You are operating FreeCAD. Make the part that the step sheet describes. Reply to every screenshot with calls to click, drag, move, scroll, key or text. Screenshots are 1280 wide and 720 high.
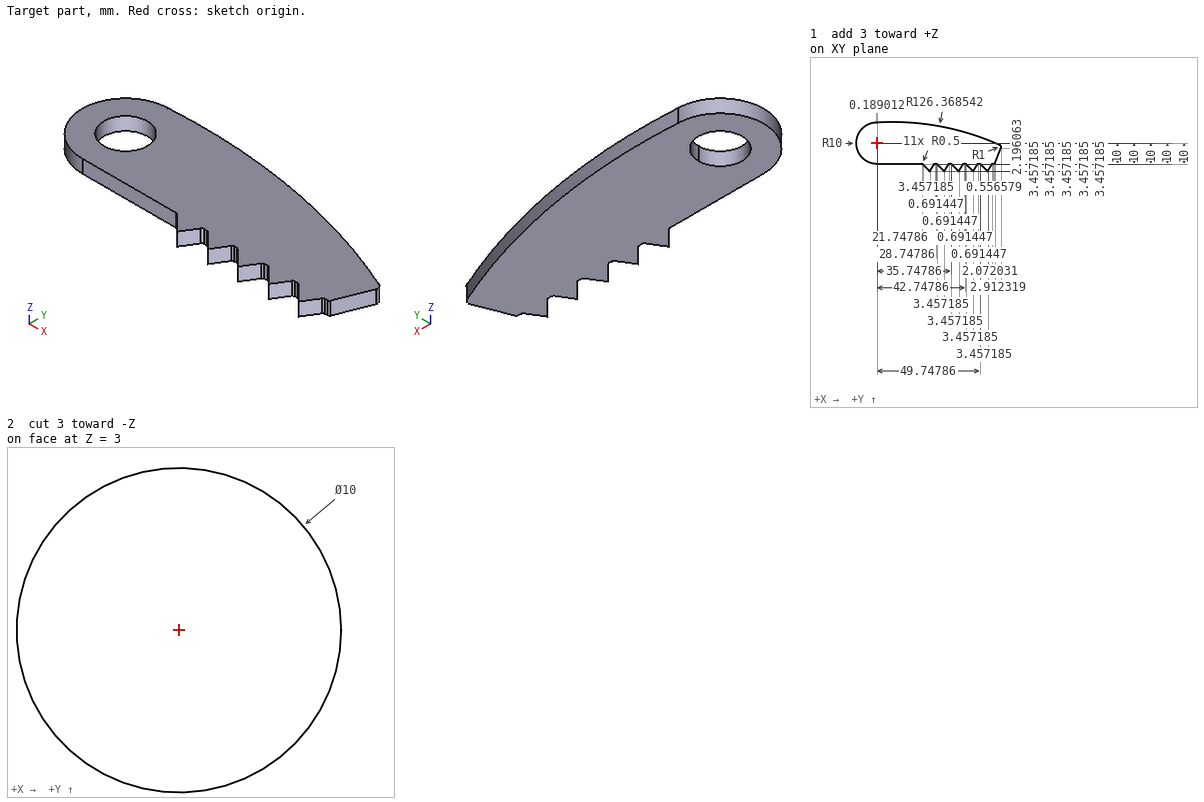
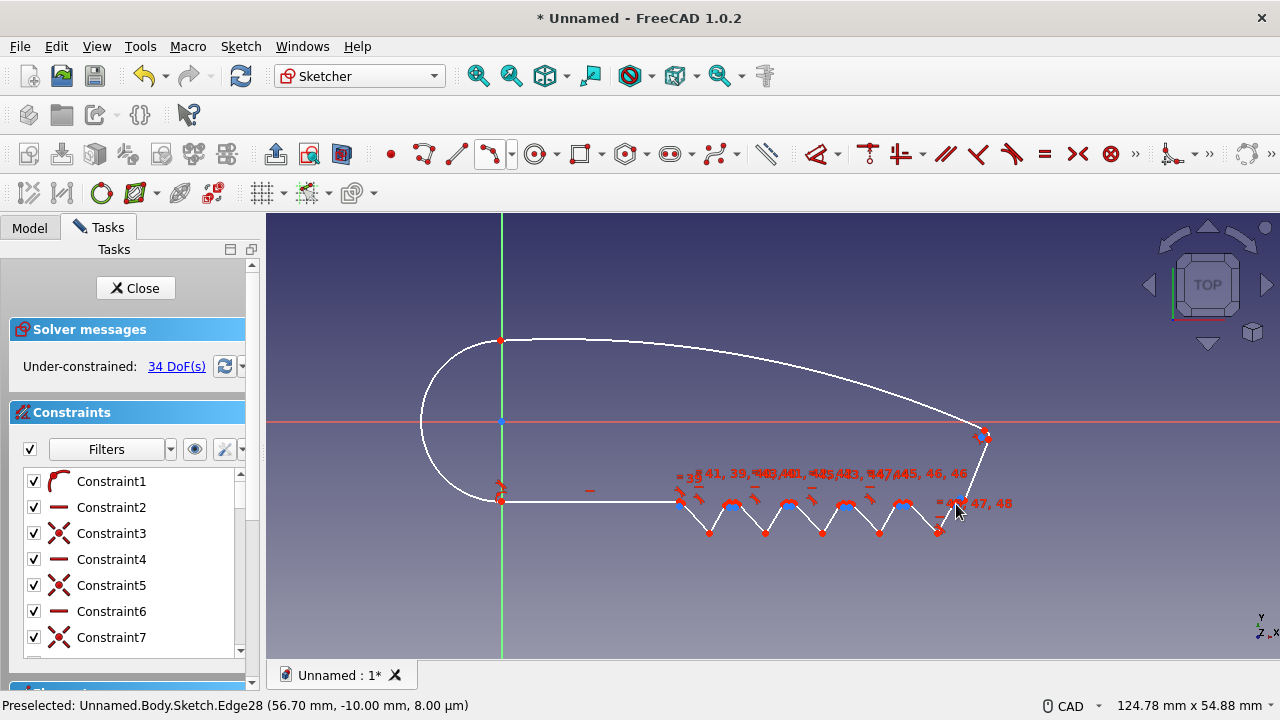
click(502, 421)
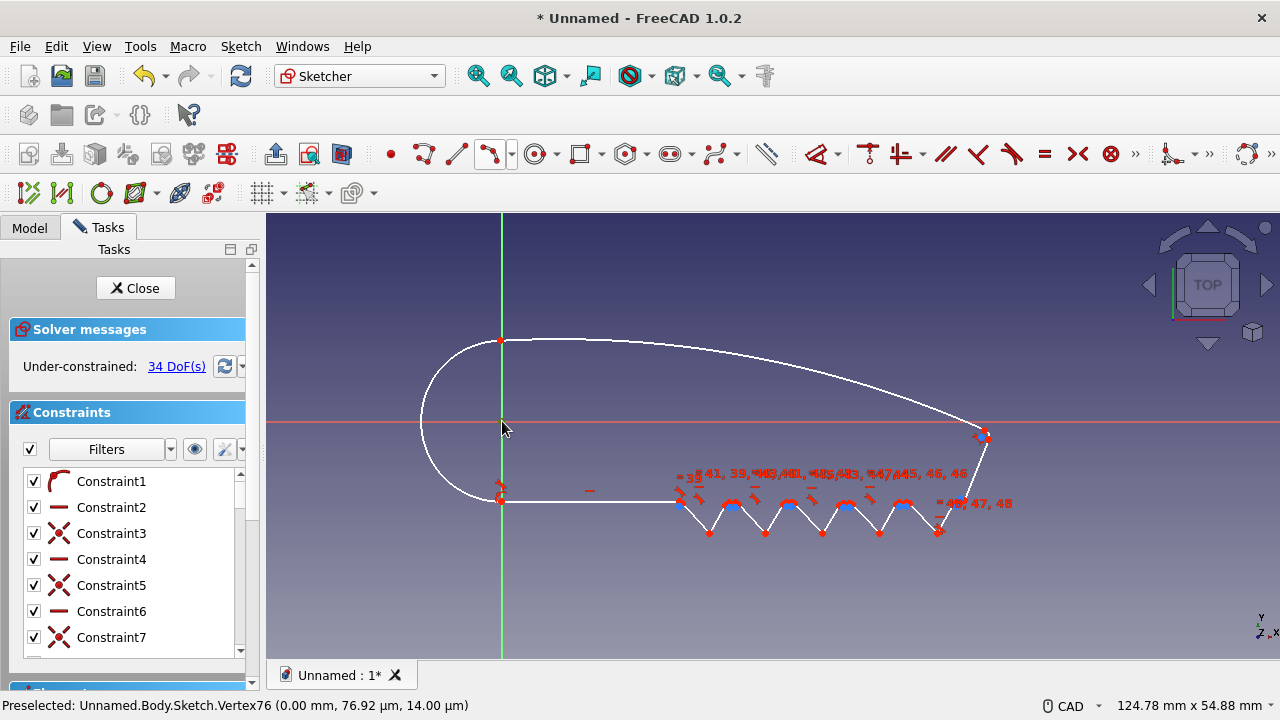
click(353, 422)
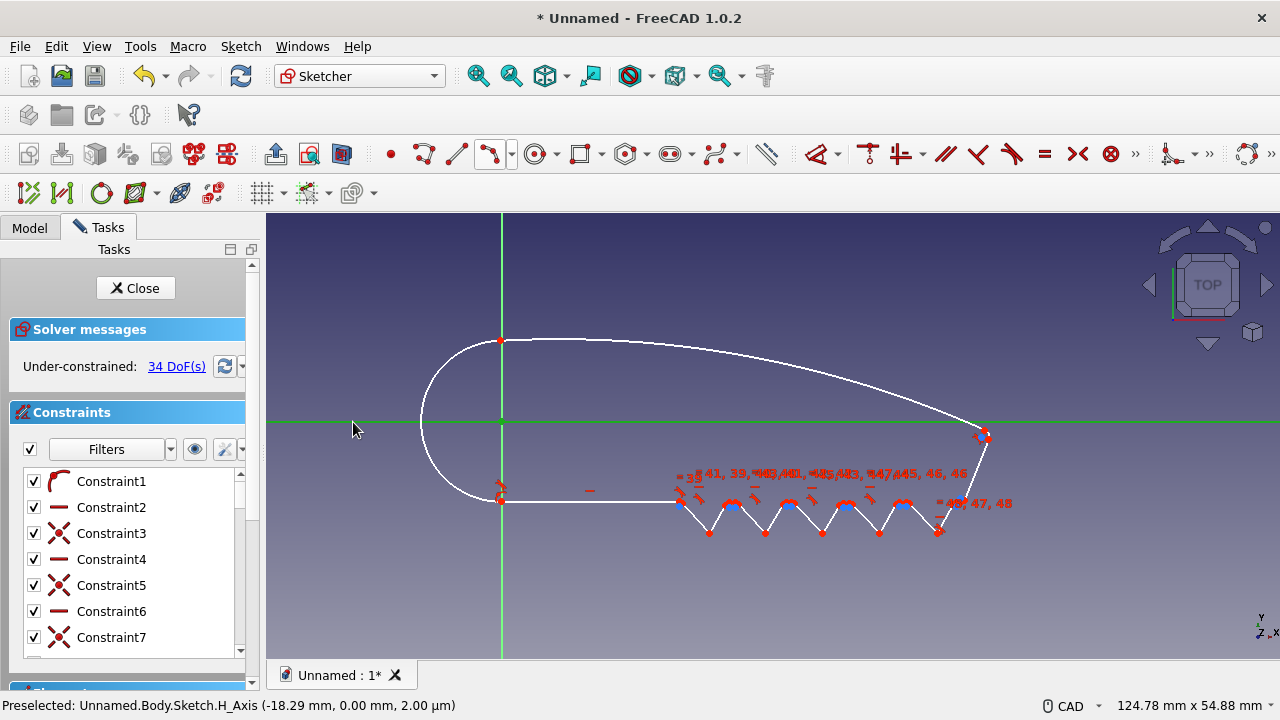
click(868, 154)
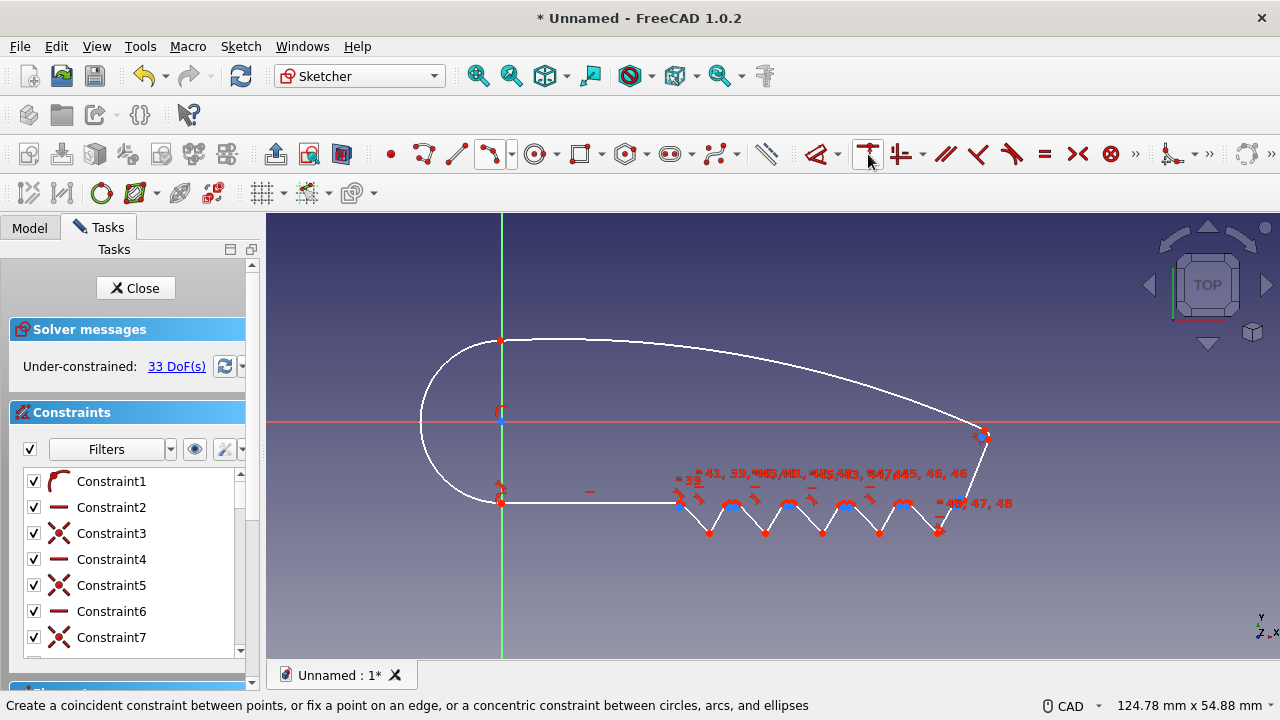
scroll(681, 503, up, 12)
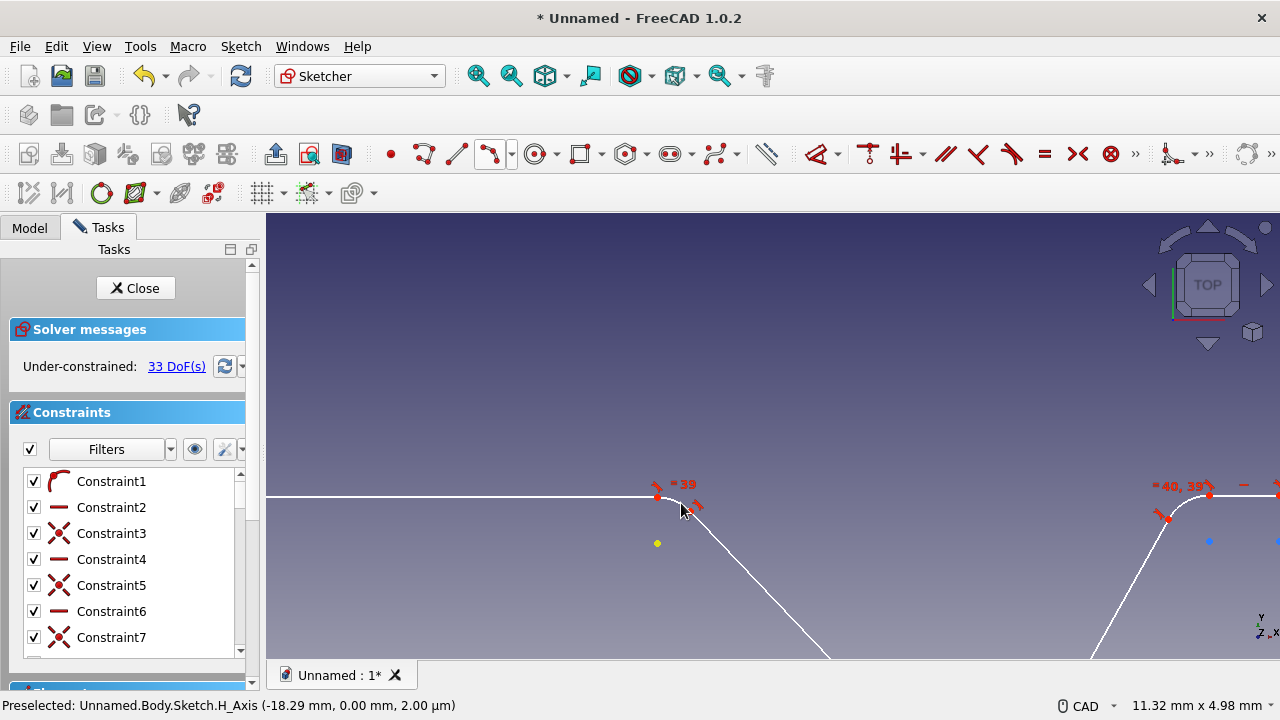
click(676, 501)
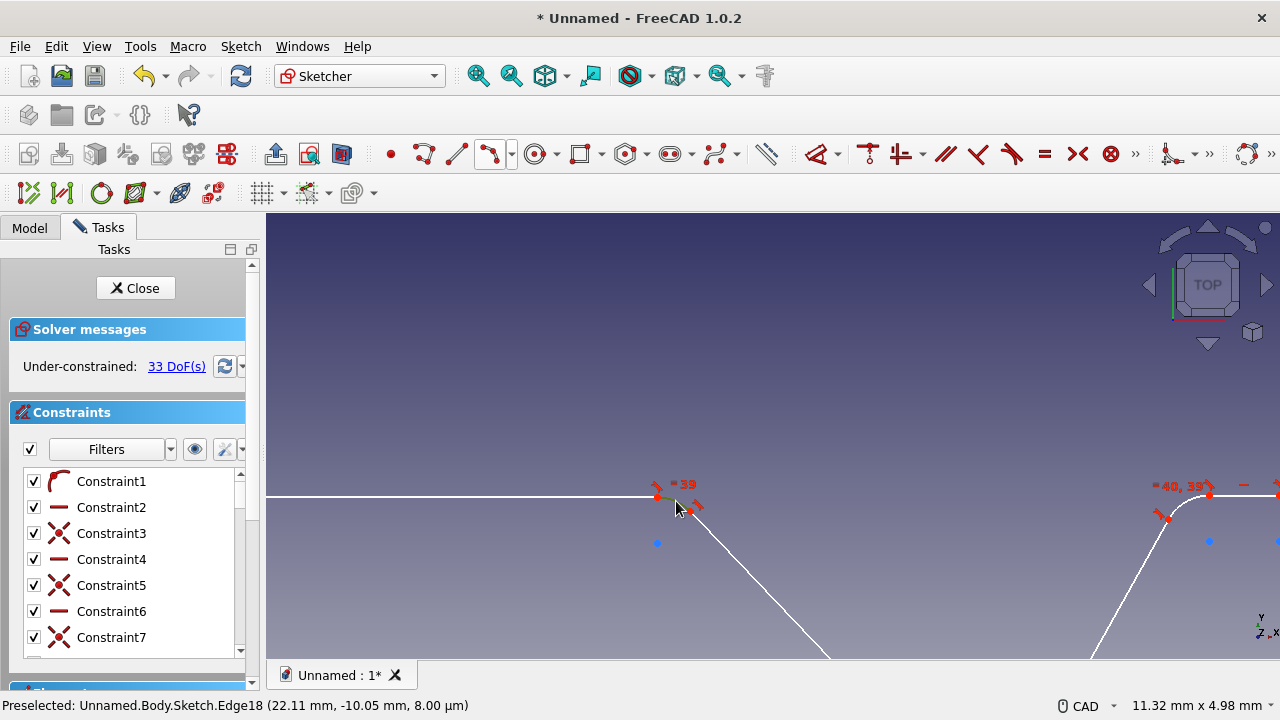
click(838, 154)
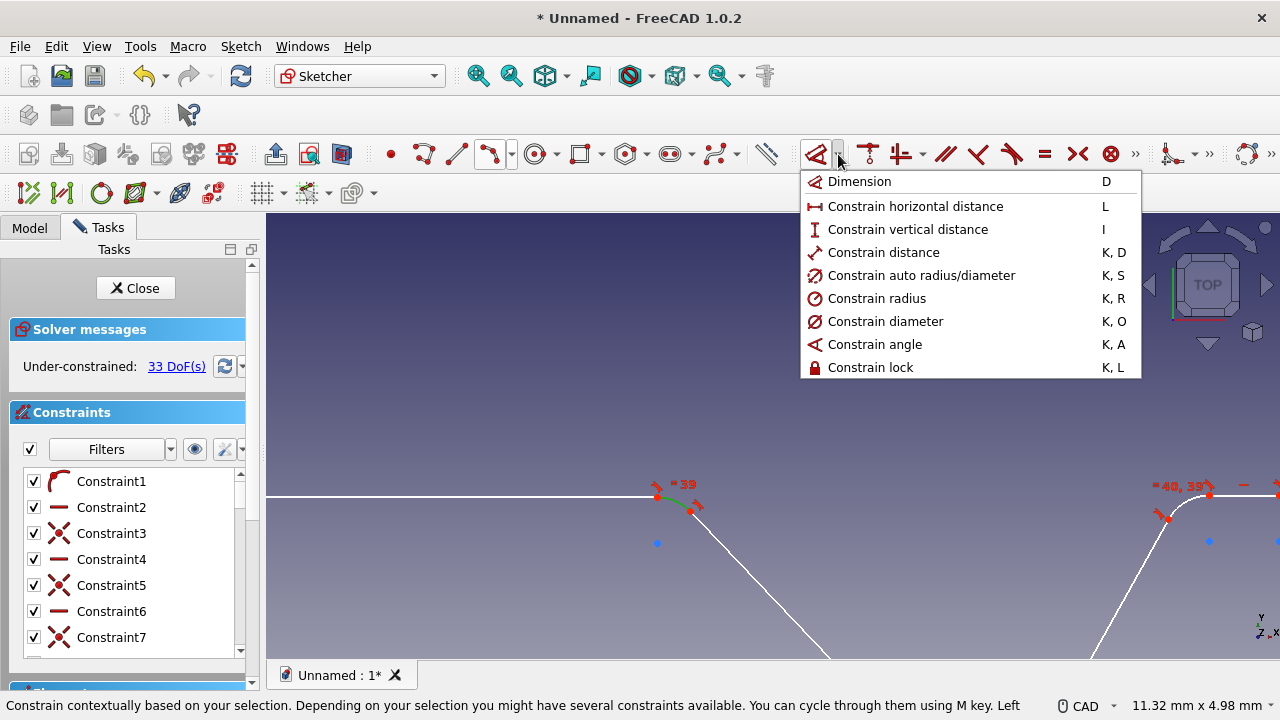
click(971, 298)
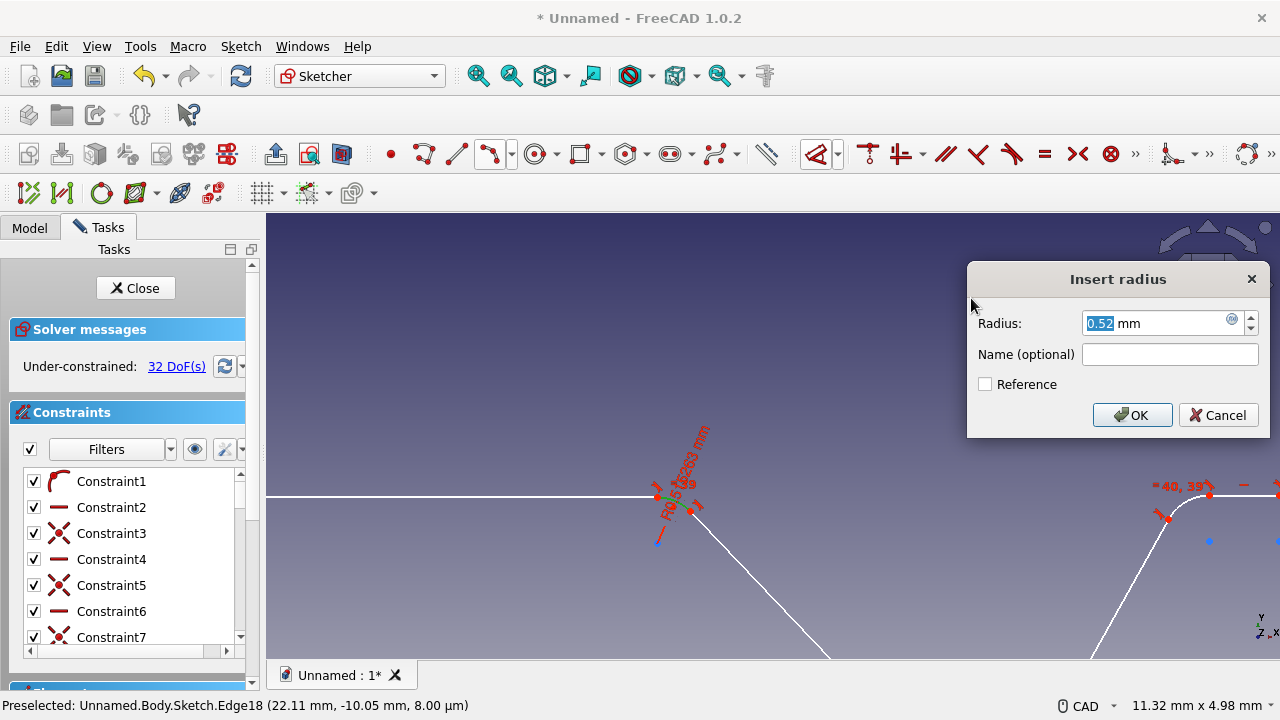
text(0.5)
key(Return)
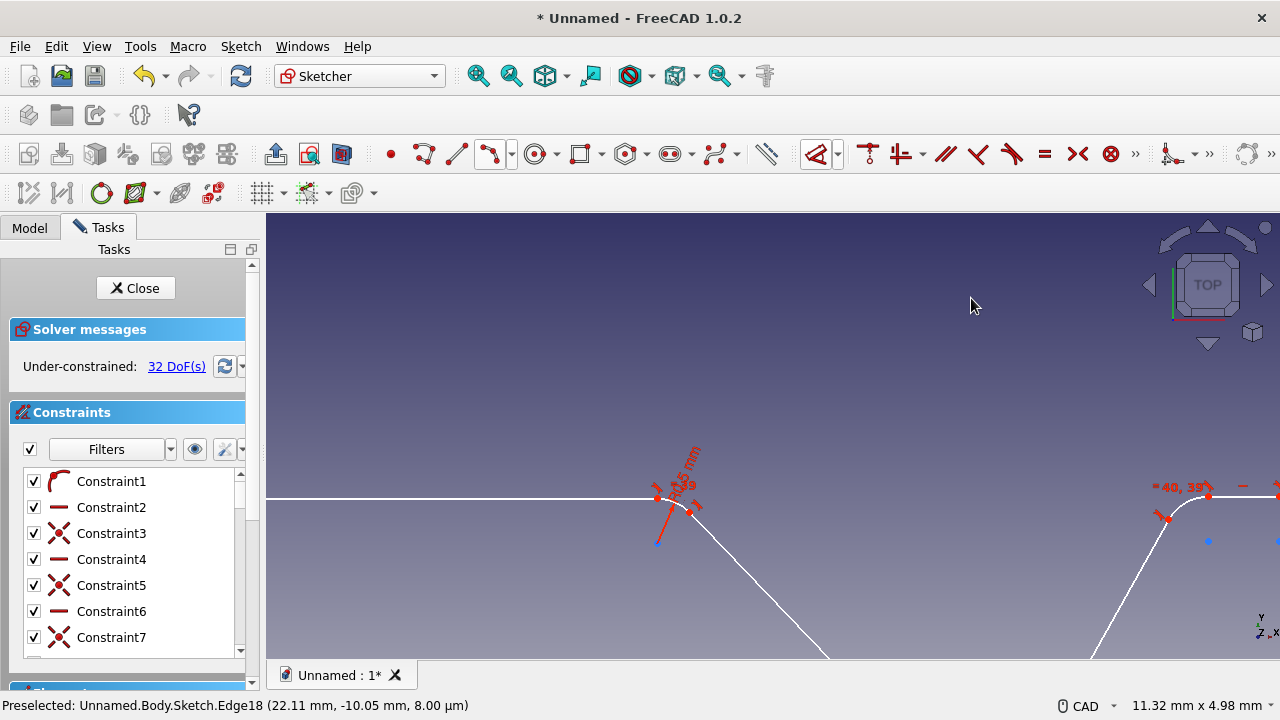
scroll(681, 503, down, 12)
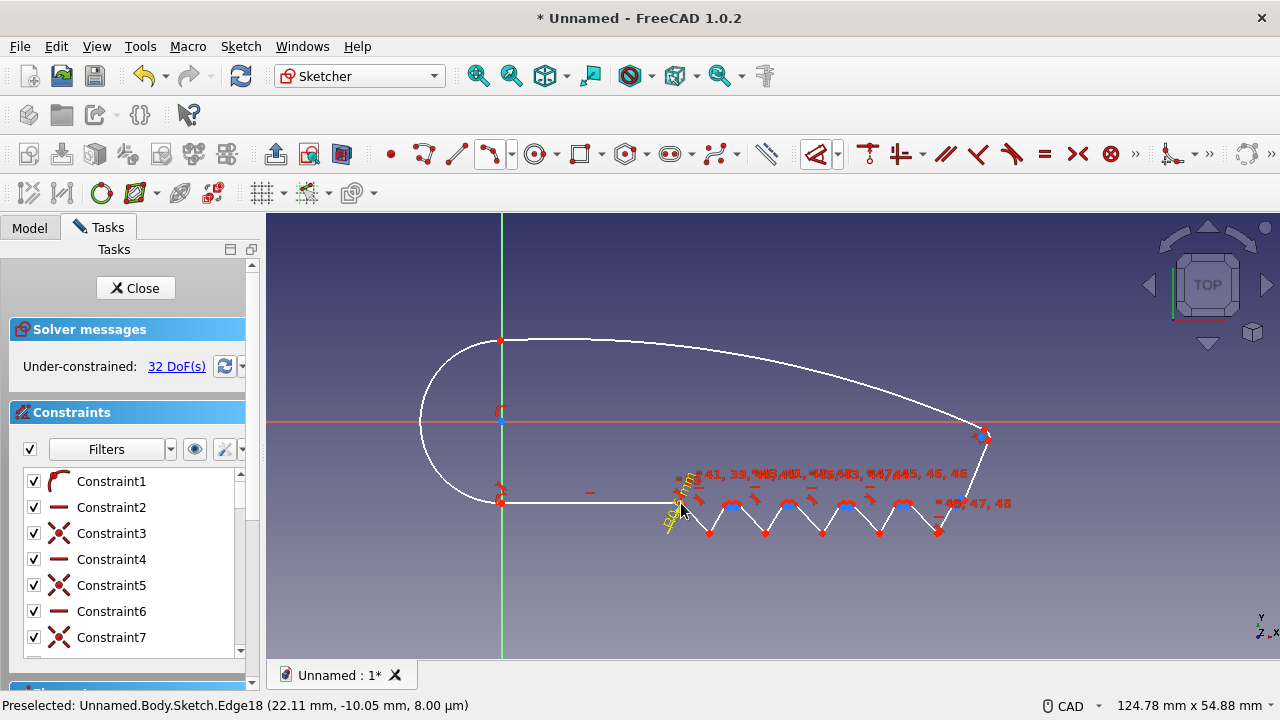
scroll(990, 436, up, 8)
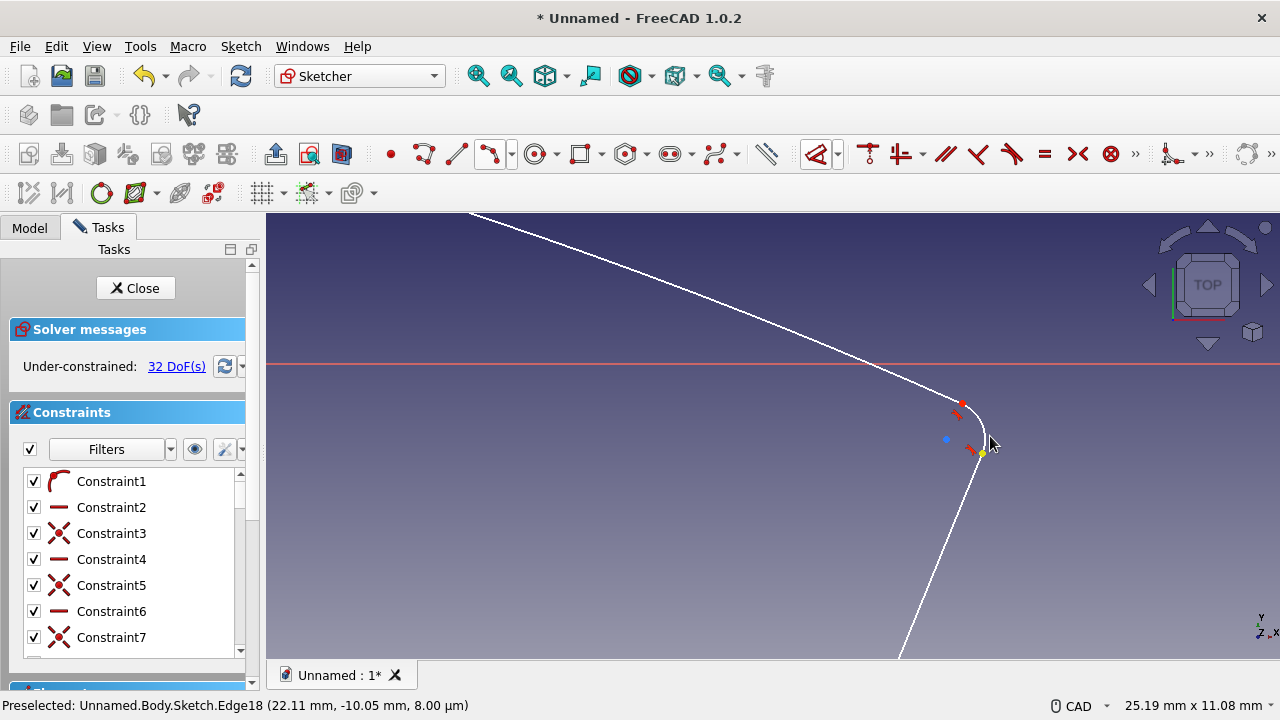
click(985, 436)